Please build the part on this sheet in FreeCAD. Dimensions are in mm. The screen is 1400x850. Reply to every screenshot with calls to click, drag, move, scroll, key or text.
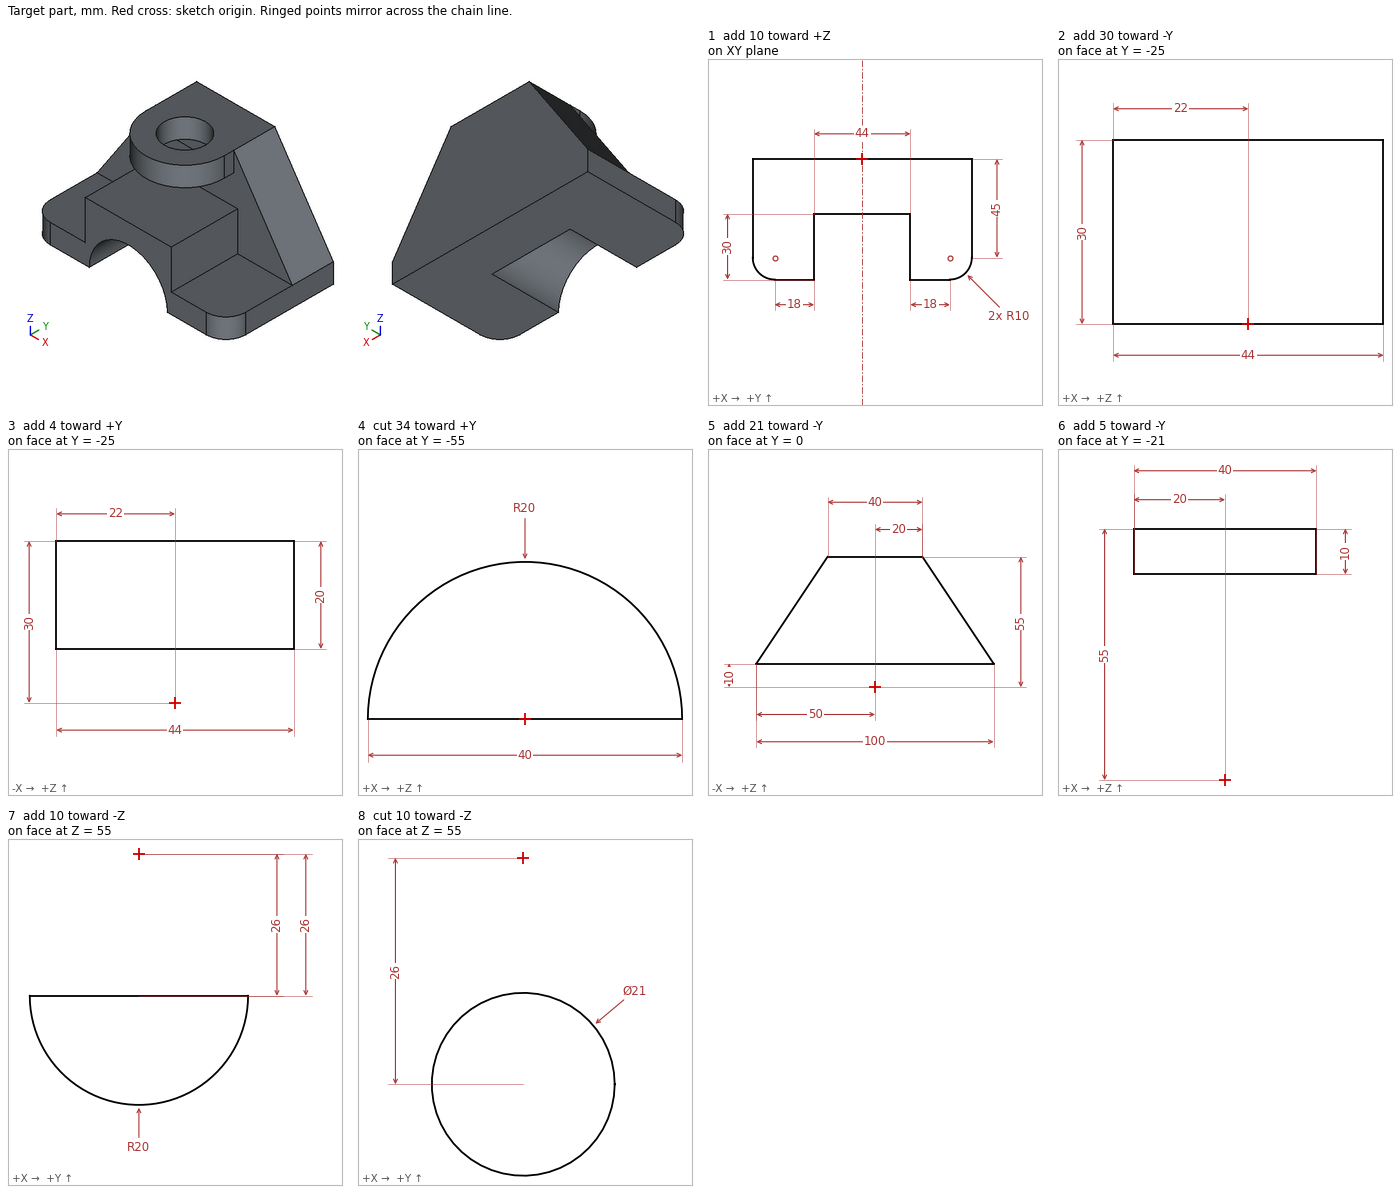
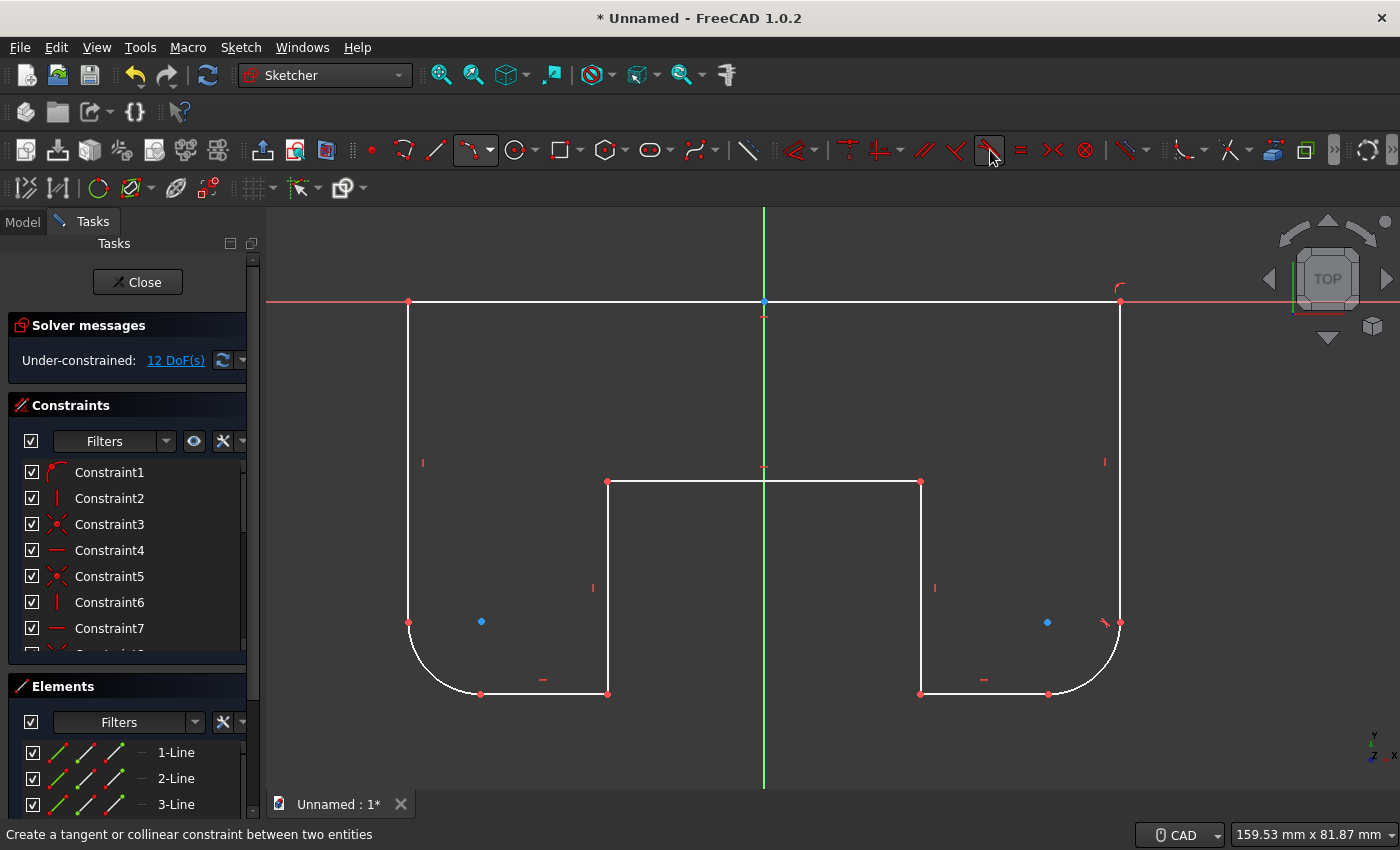
click(408, 398)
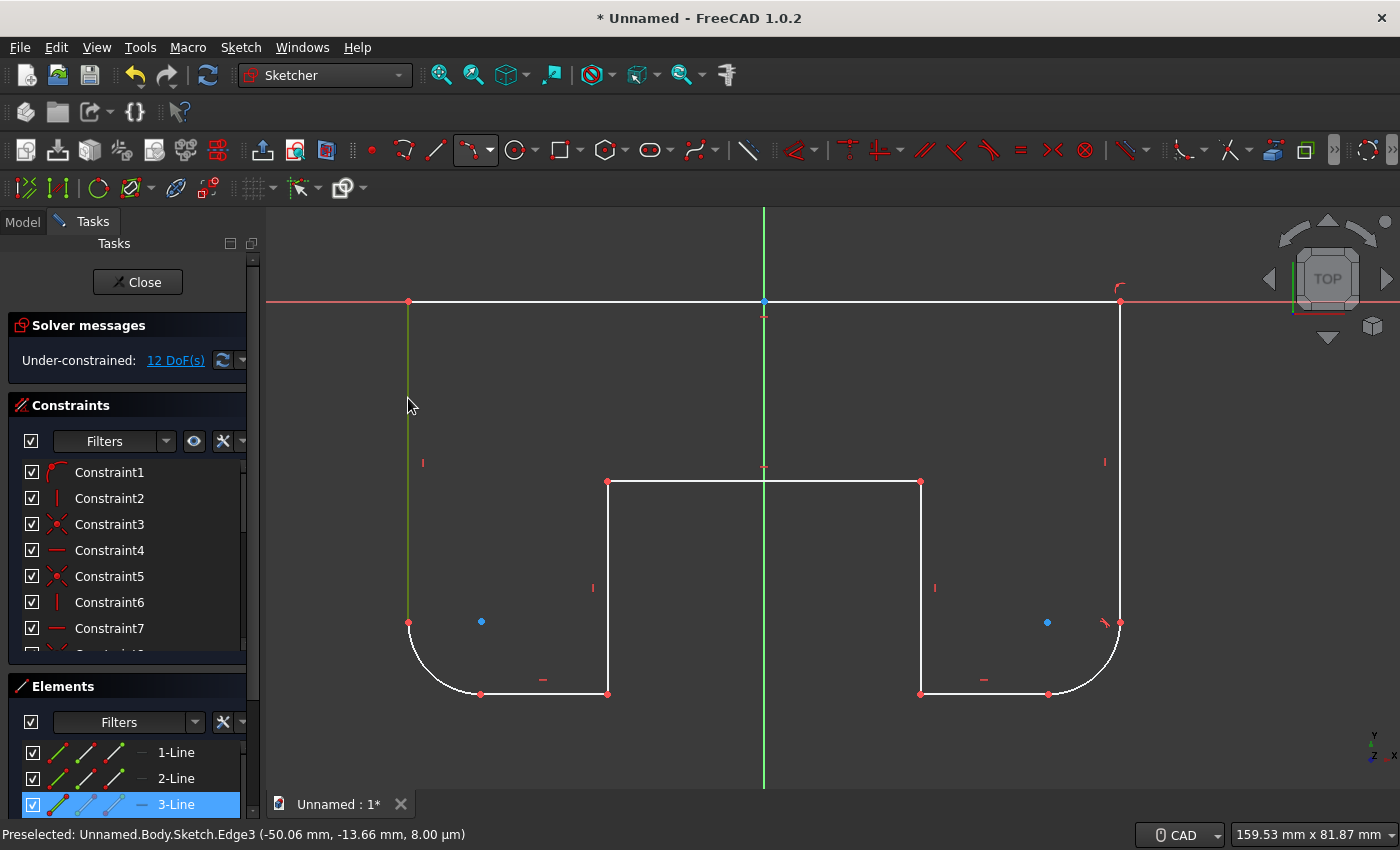
click(417, 655)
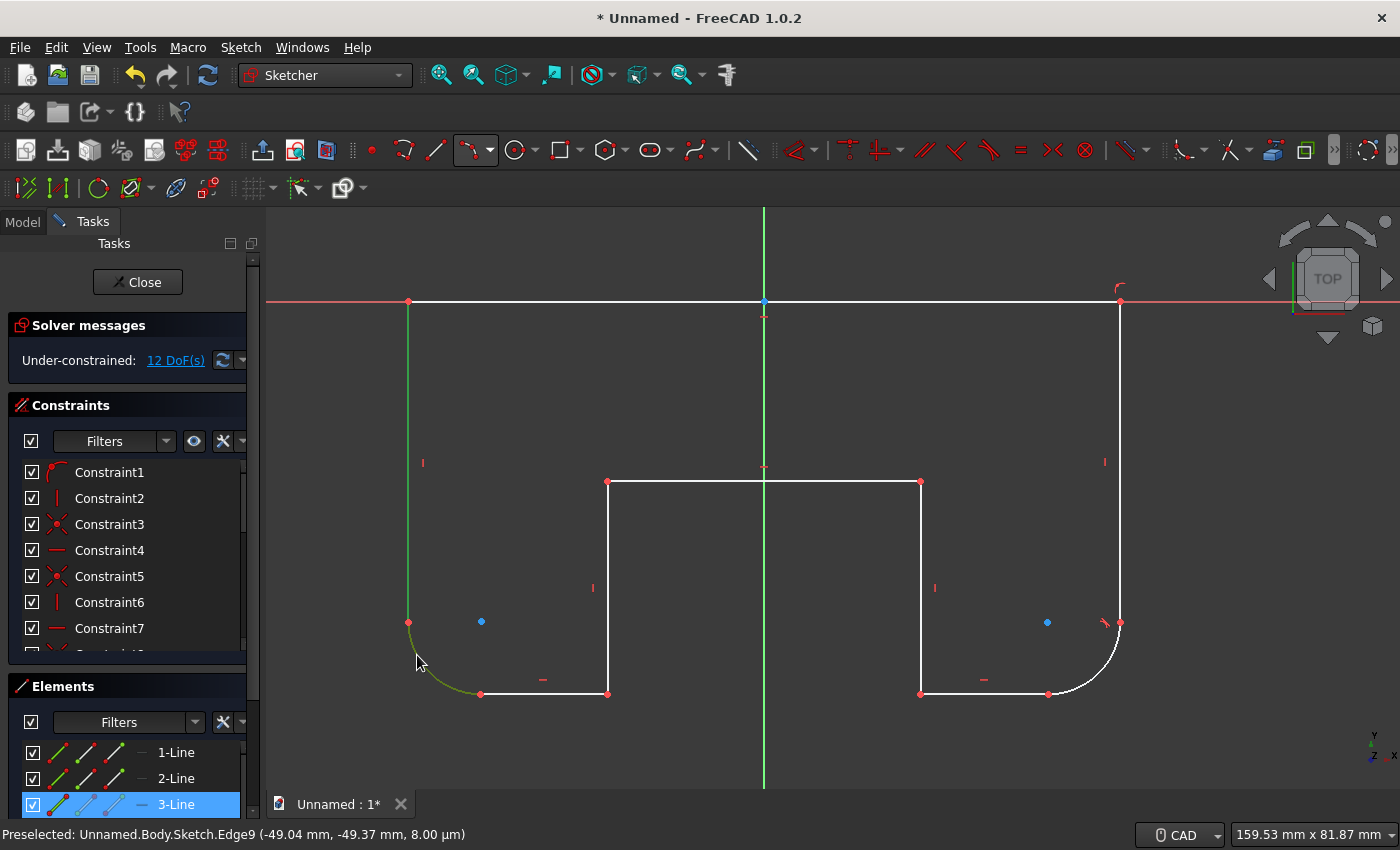
click(990, 150)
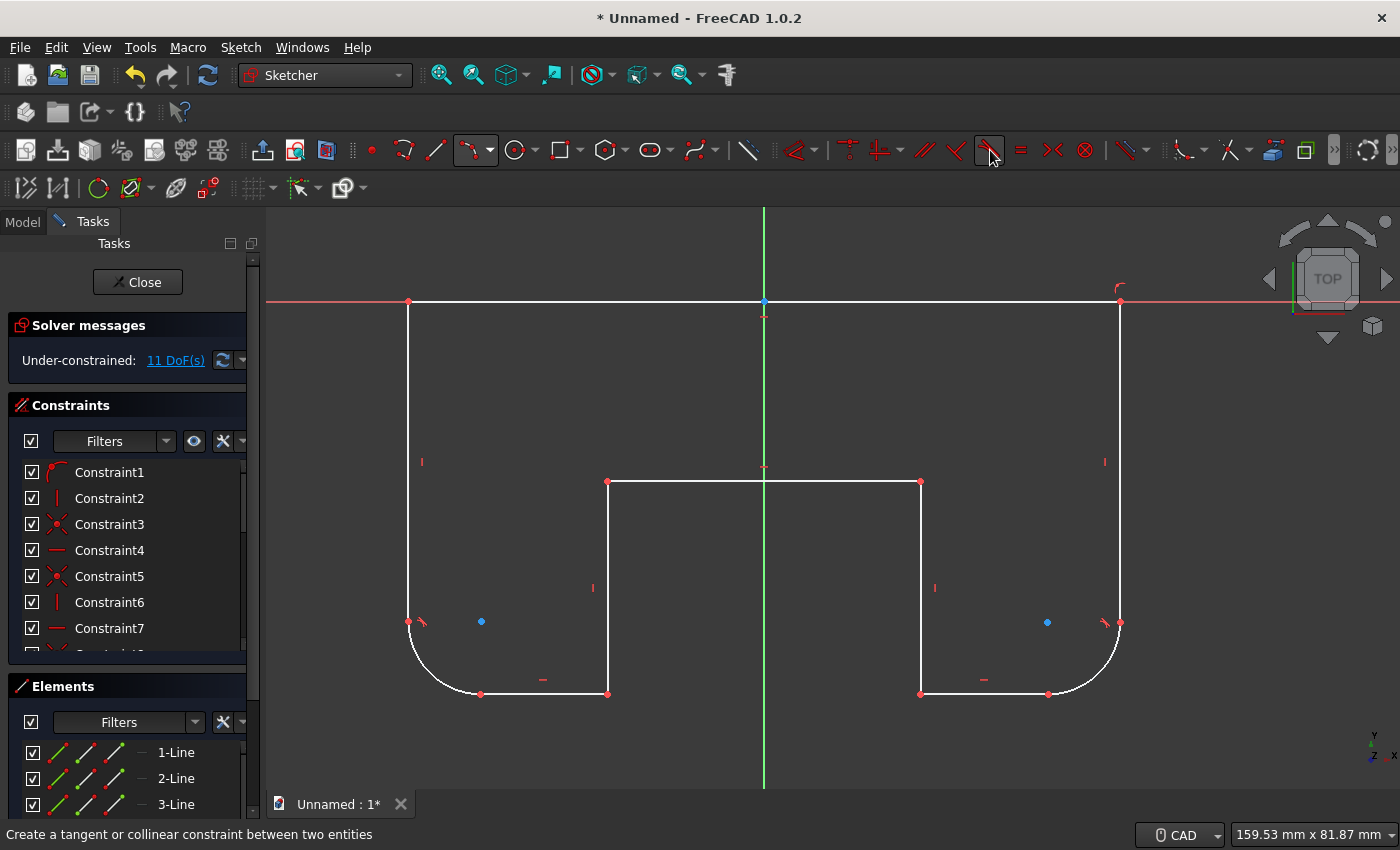
click(518, 694)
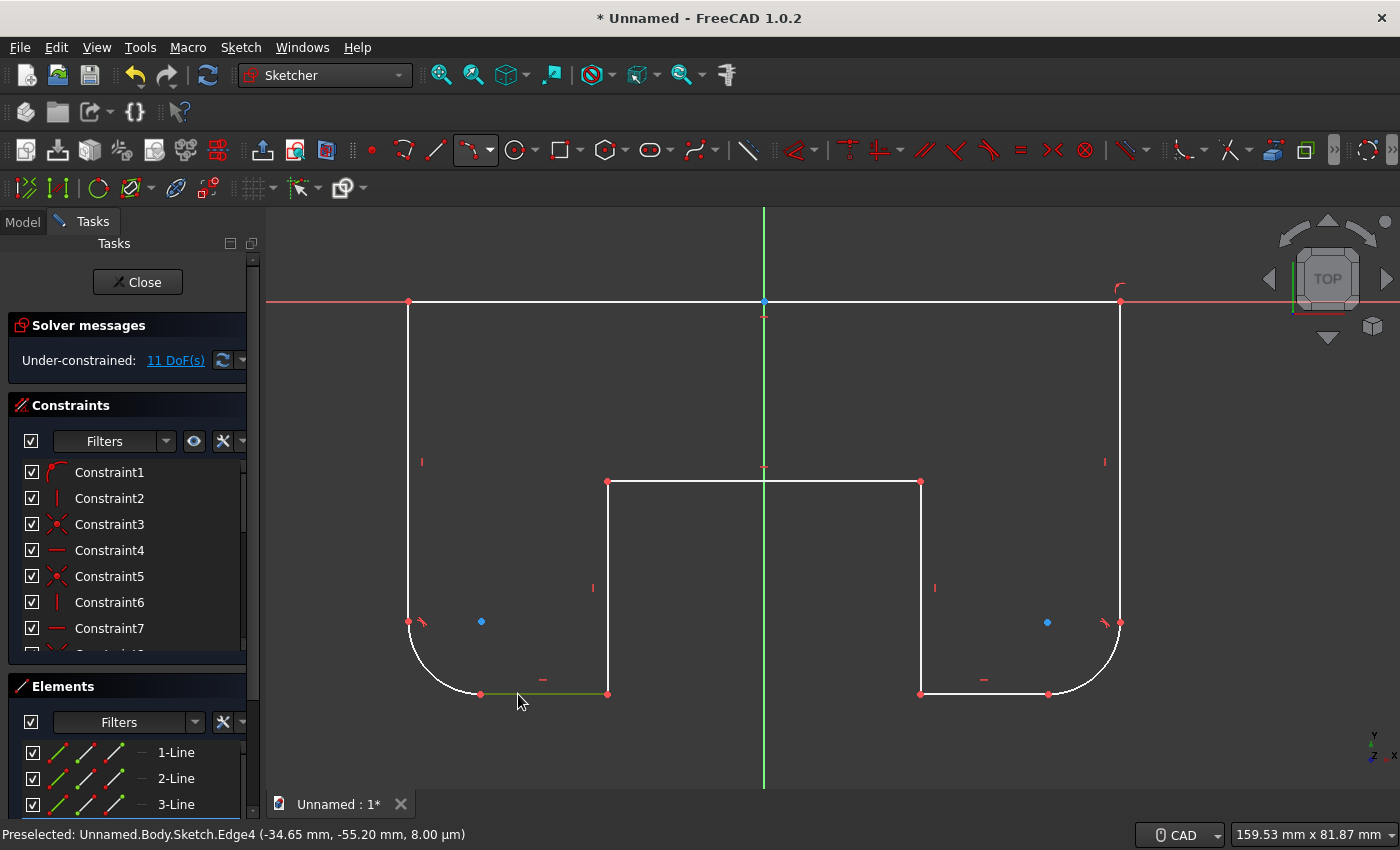
click(416, 654)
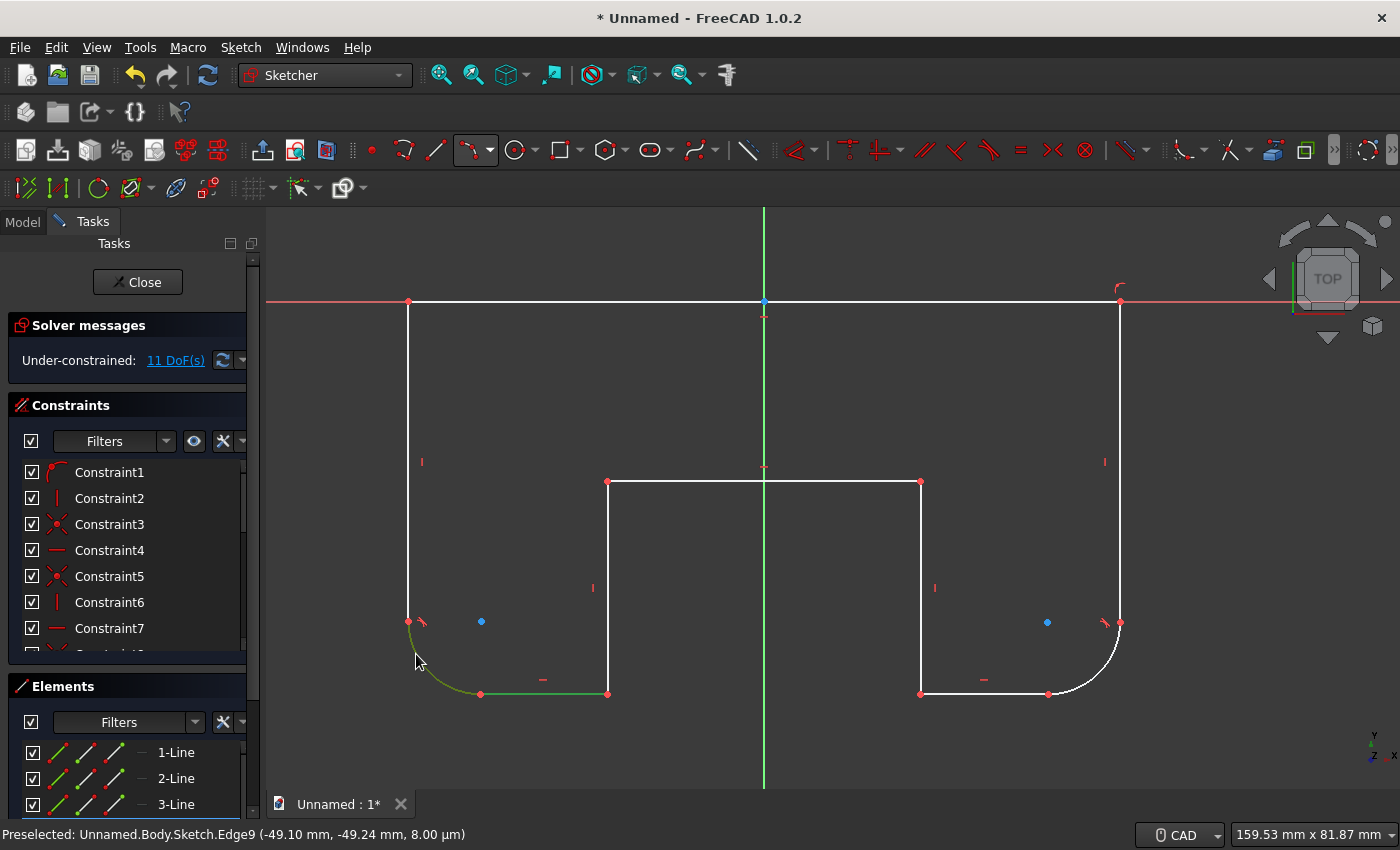
click(990, 150)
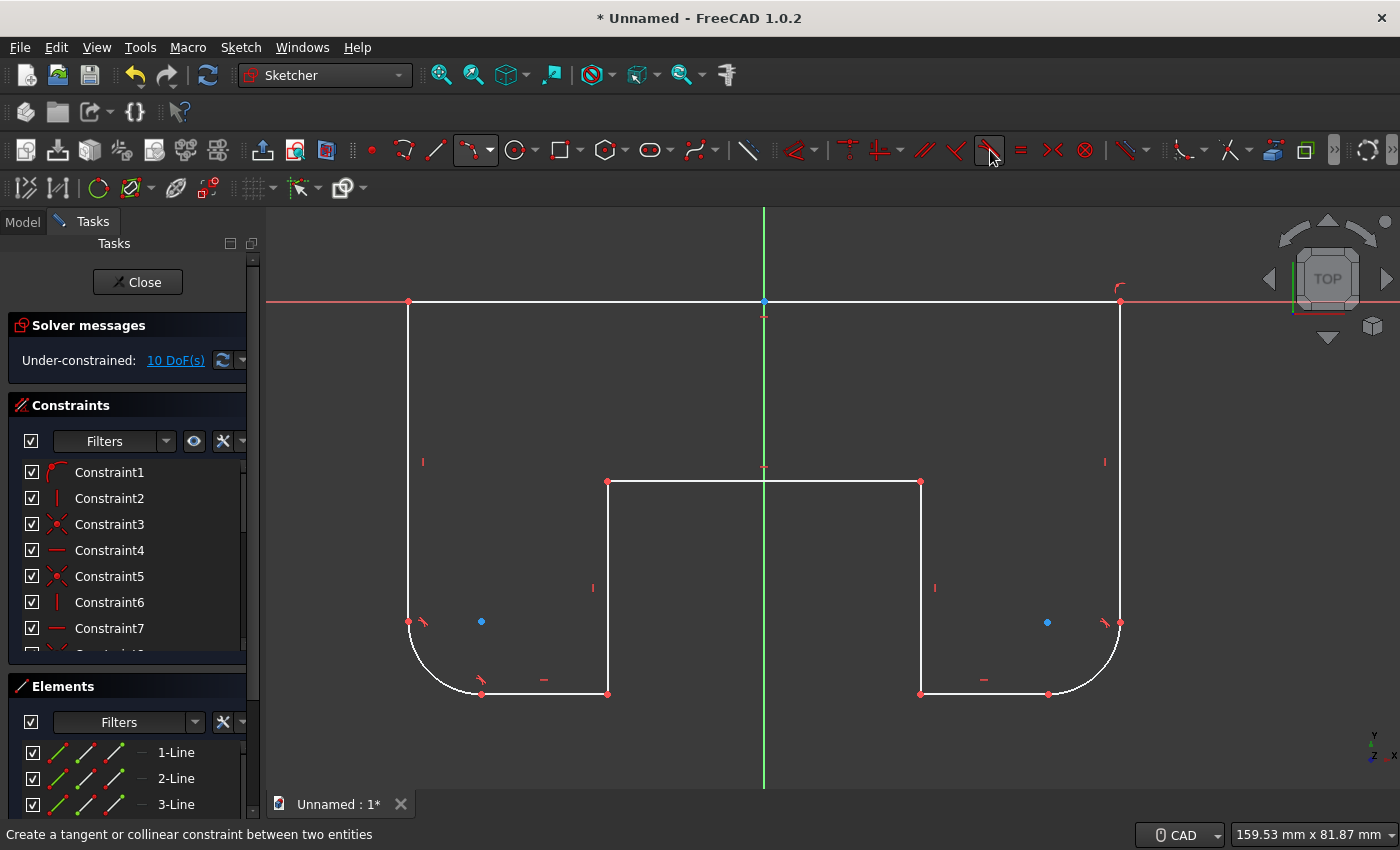
click(959, 694)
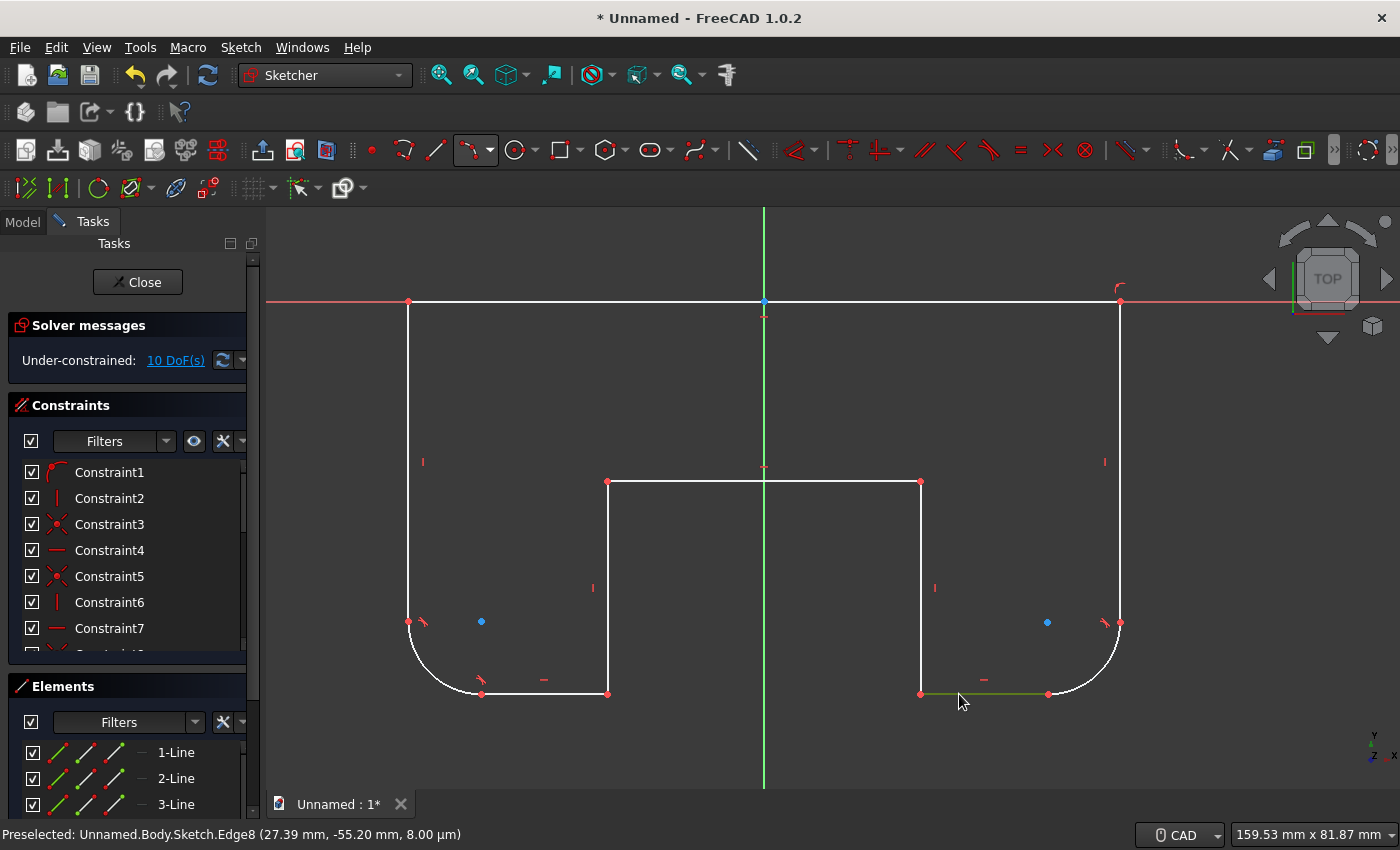
click(1081, 686)